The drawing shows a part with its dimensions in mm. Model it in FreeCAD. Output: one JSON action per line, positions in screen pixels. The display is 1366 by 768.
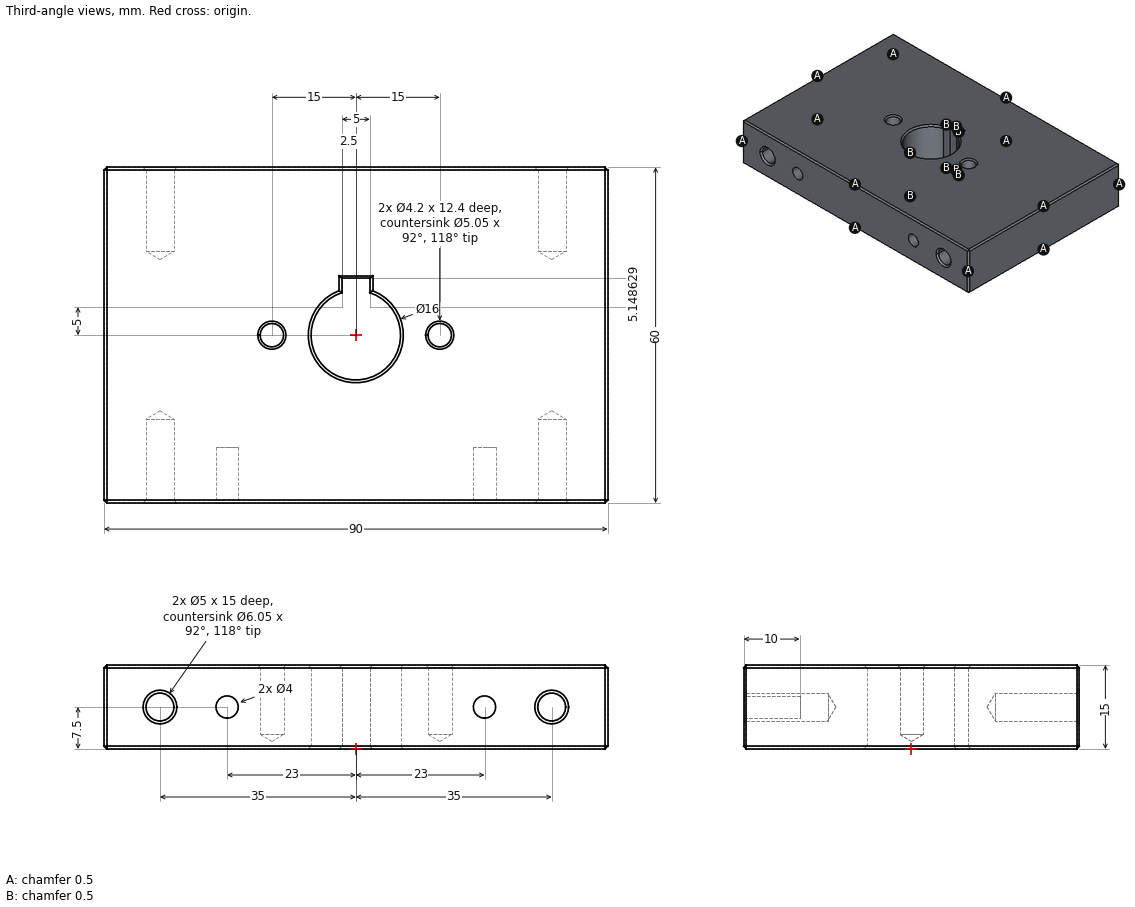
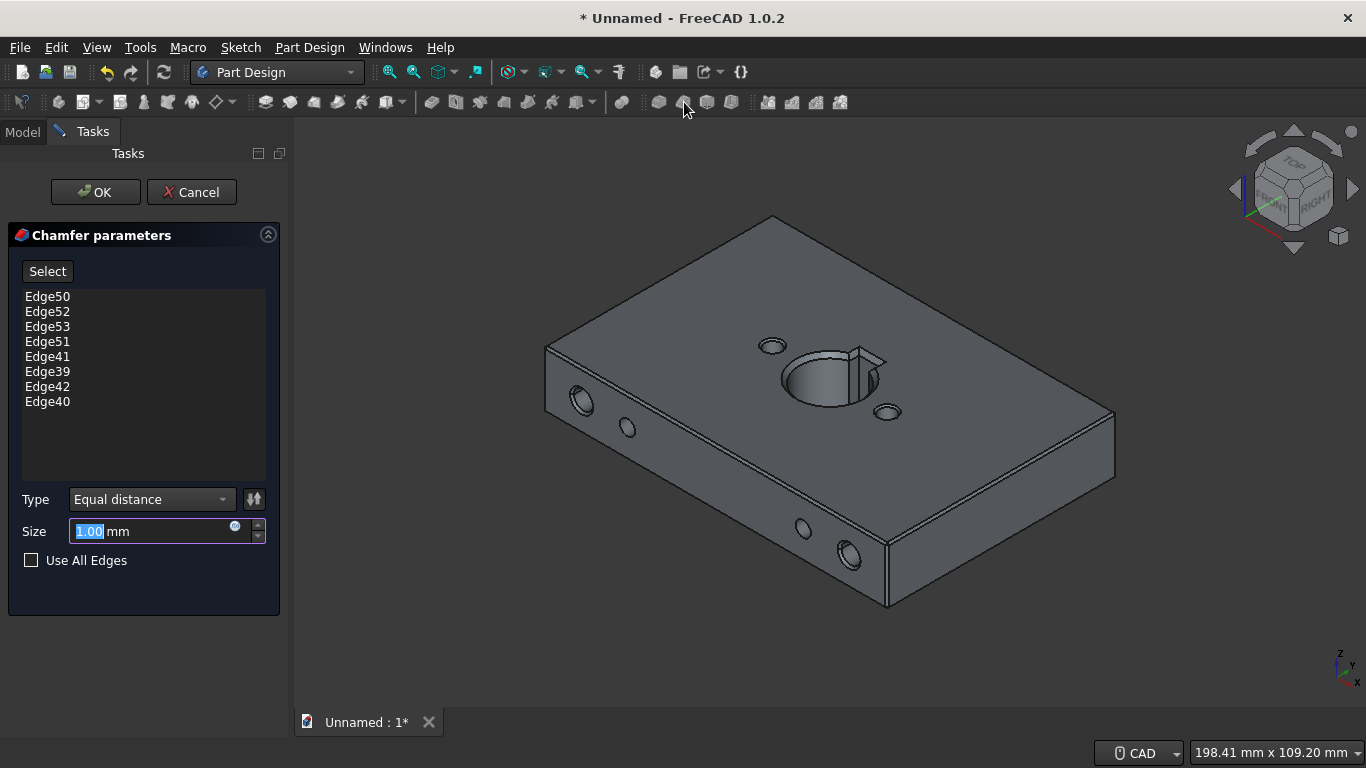
{"action": "type", "text": "0.5"}
{"action": "key", "text": "Tab"}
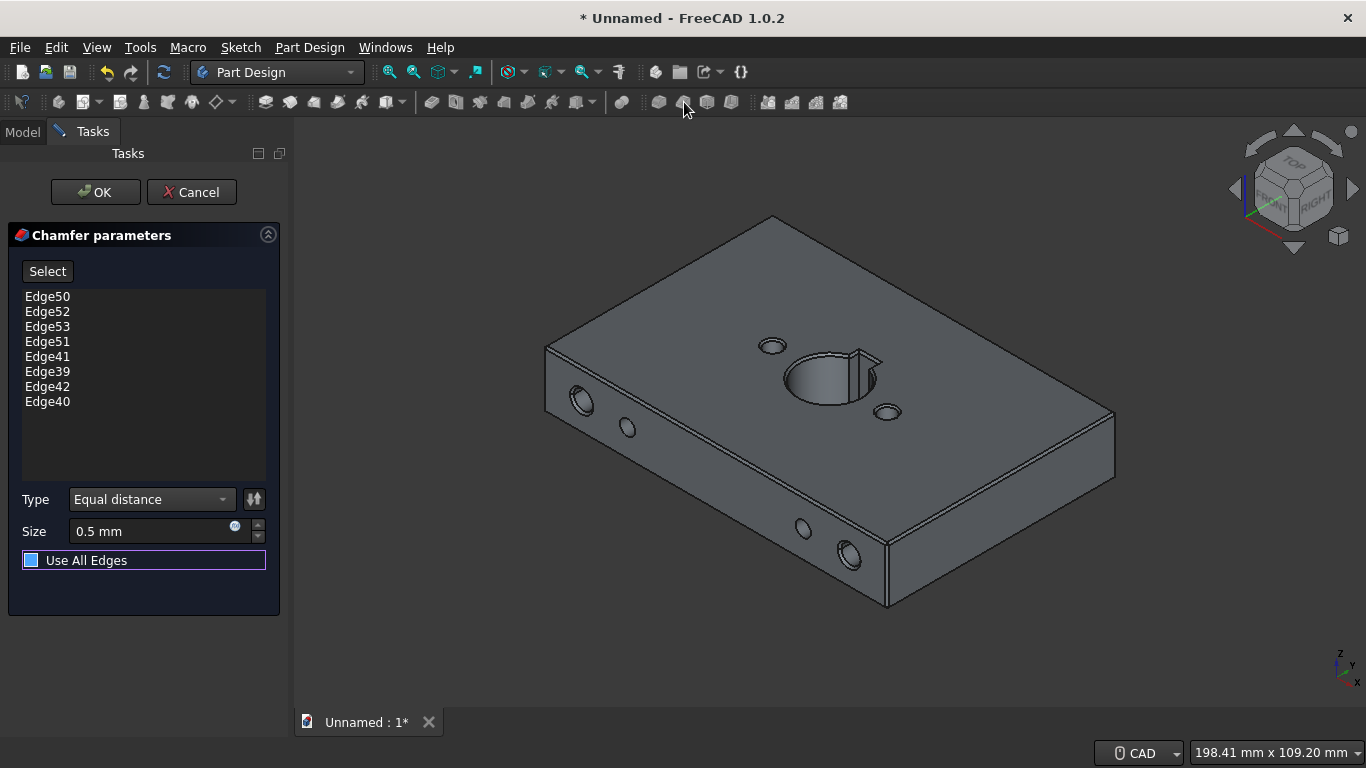
{"action": "left_click", "coordinate": [96, 192]}